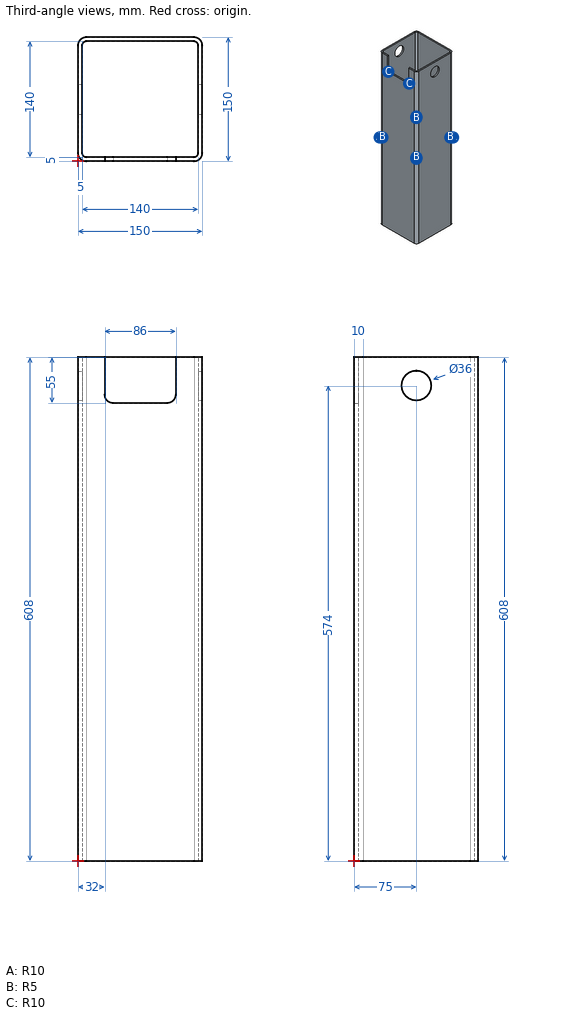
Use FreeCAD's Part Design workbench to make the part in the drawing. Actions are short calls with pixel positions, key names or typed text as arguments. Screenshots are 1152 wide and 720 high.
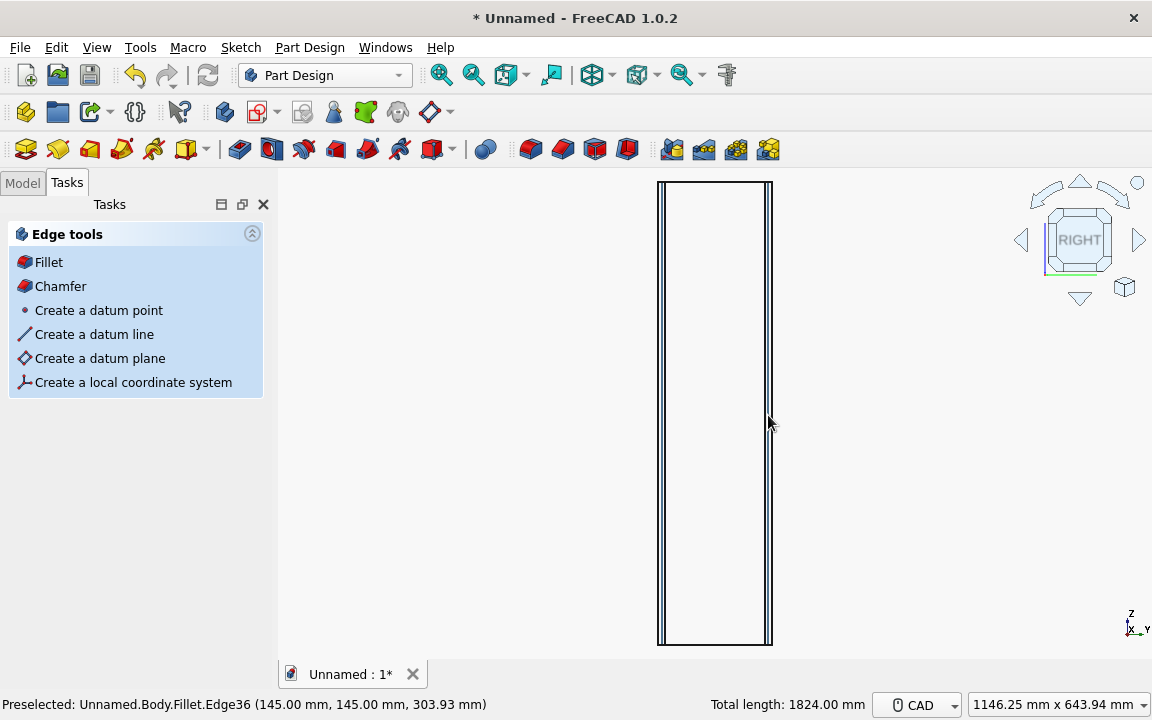
key(5)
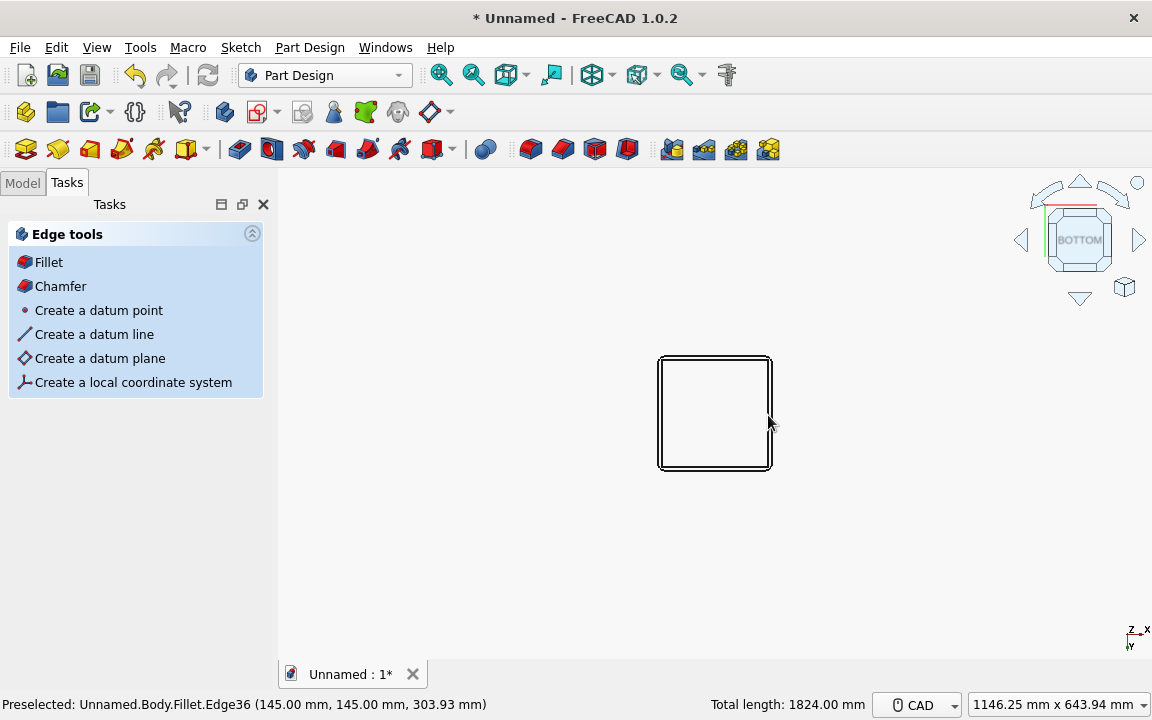
key(v)
key(f)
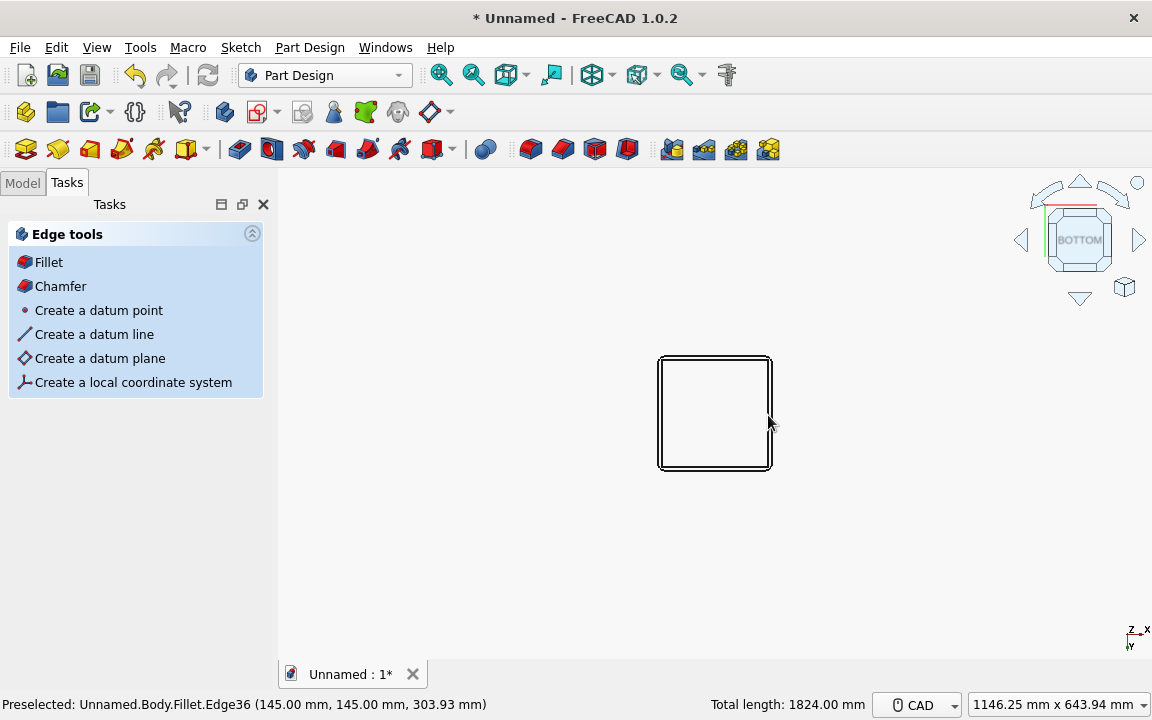
scroll(662, 466, up, 6)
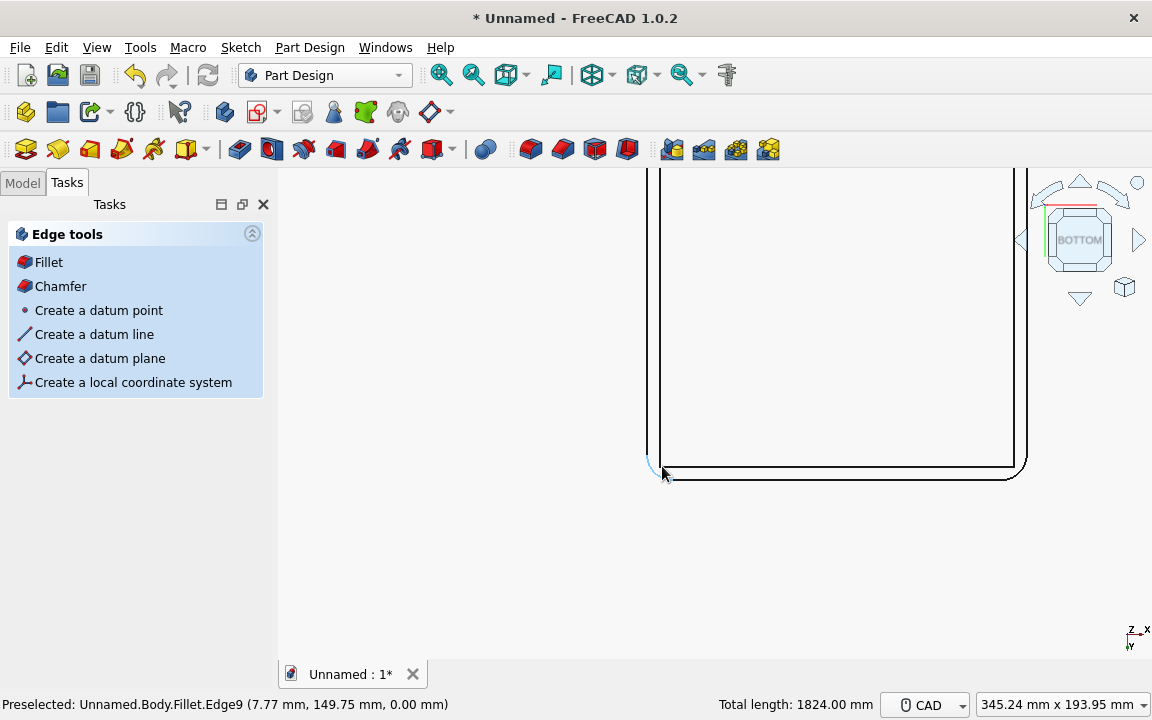
key(v)
key(f)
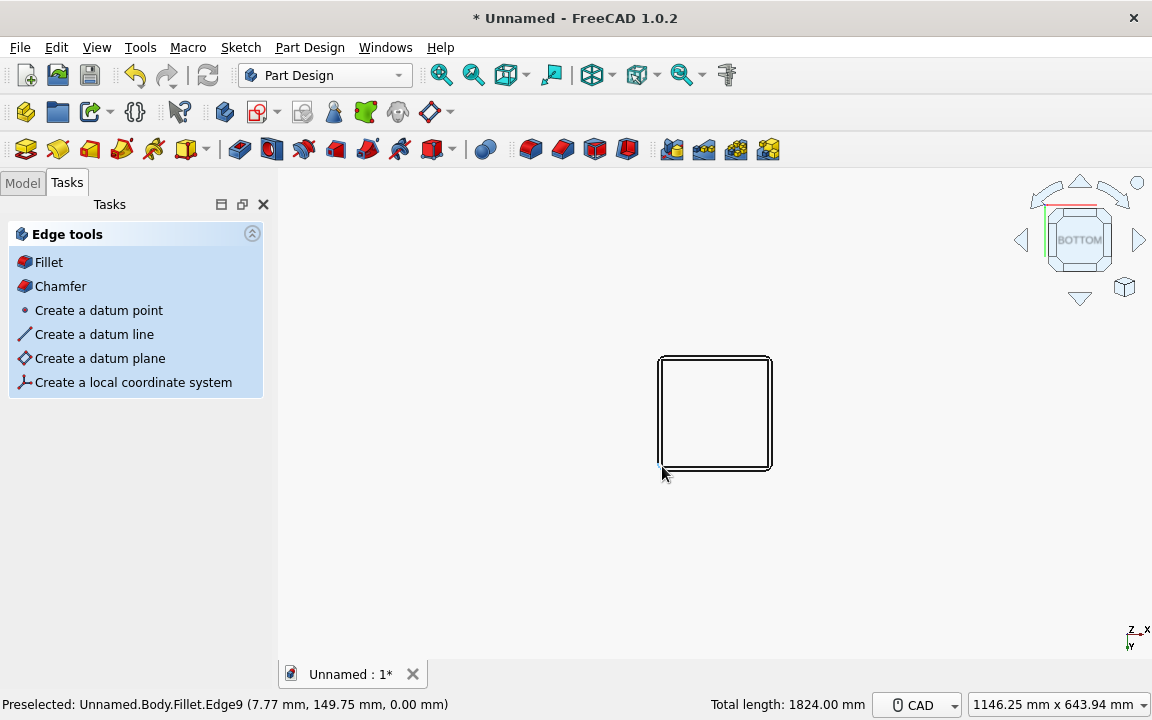
key(4)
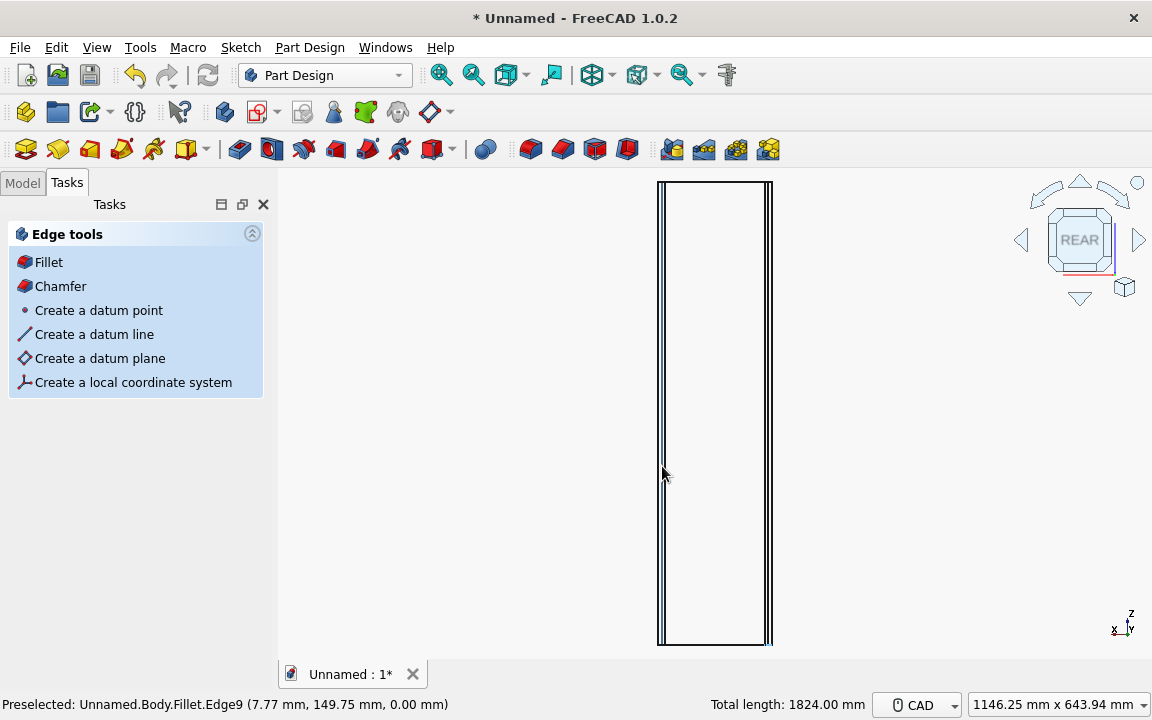
scroll(768, 413, up, 6)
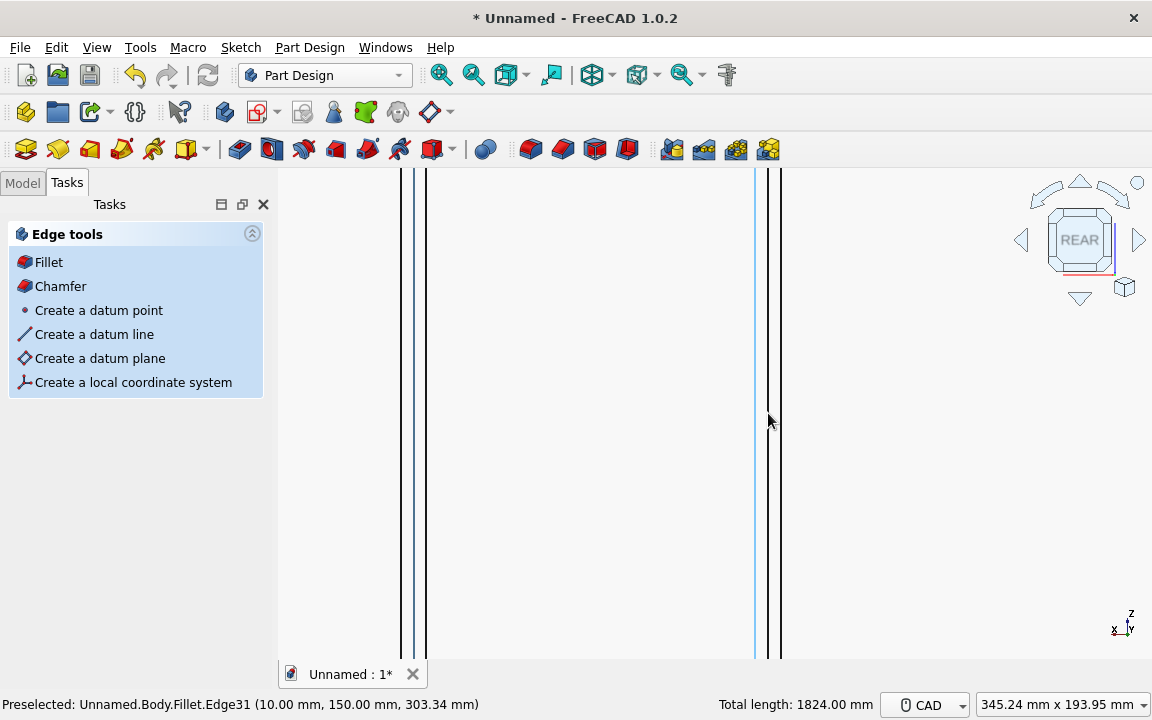
click(768, 413, ctrl)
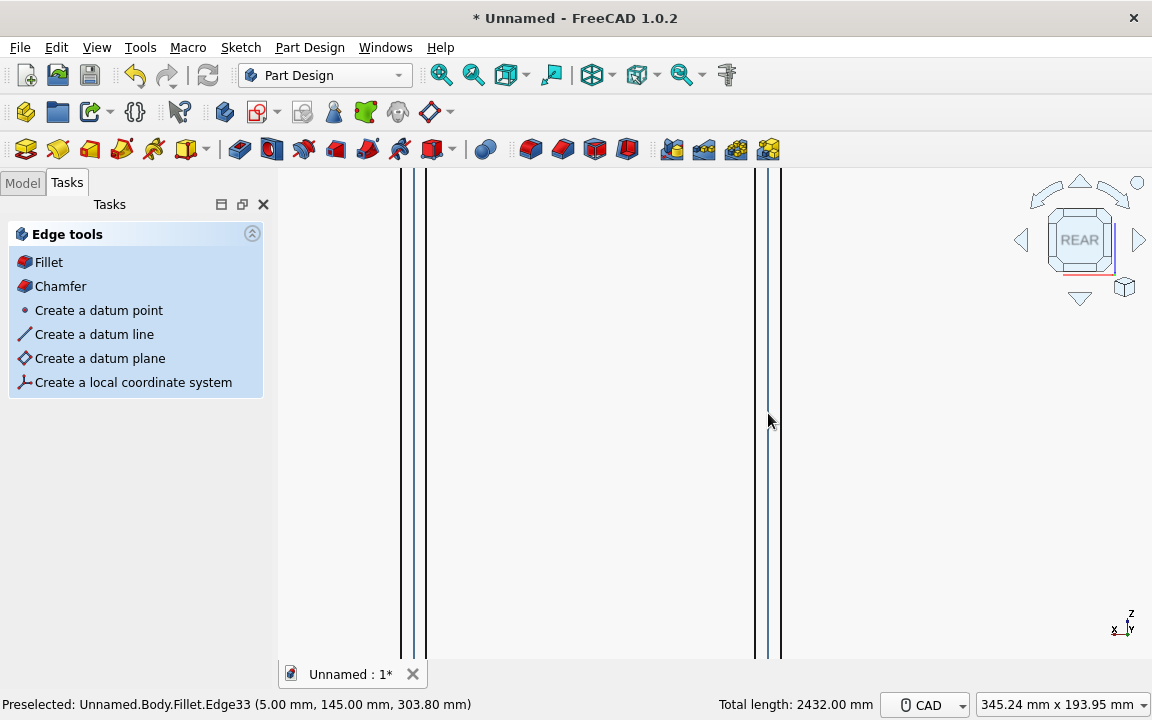
key(v)
key(1)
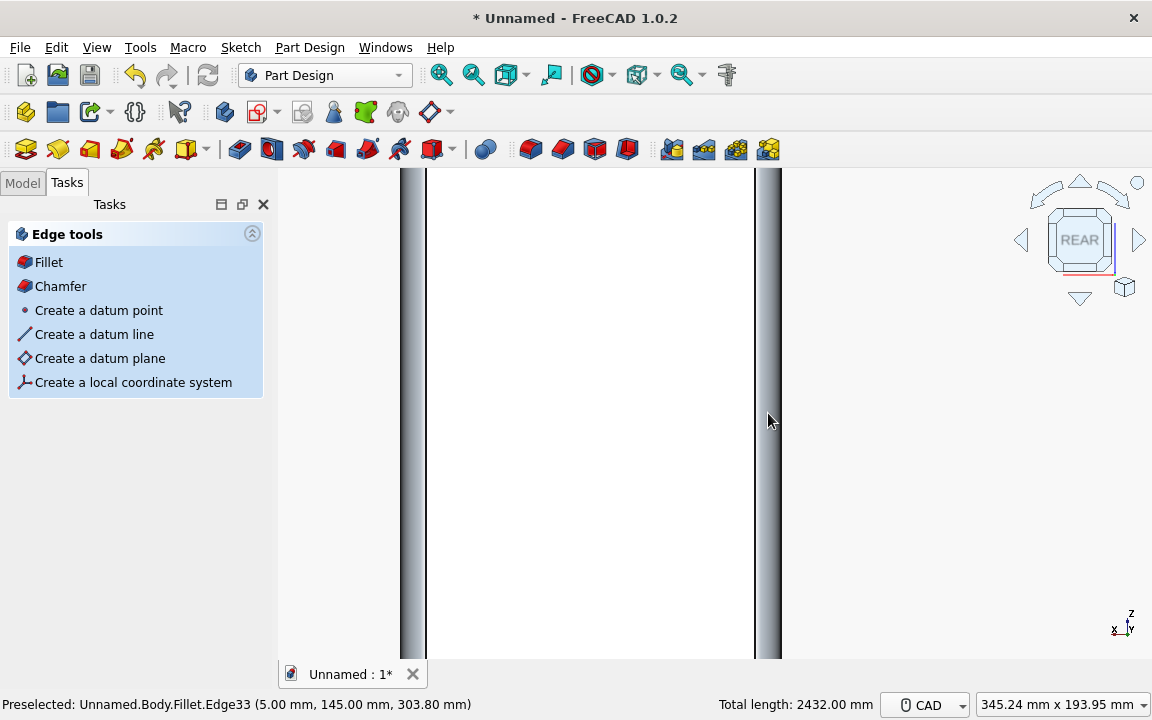
click(532, 150)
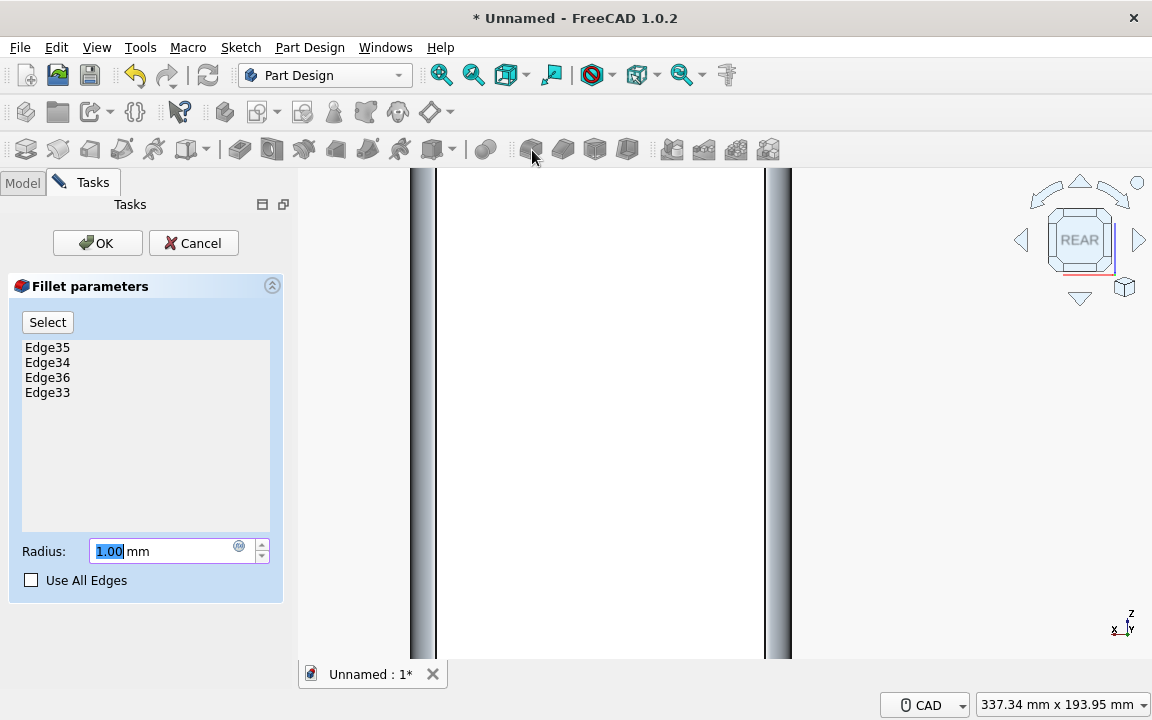
text(5)
key(Tab)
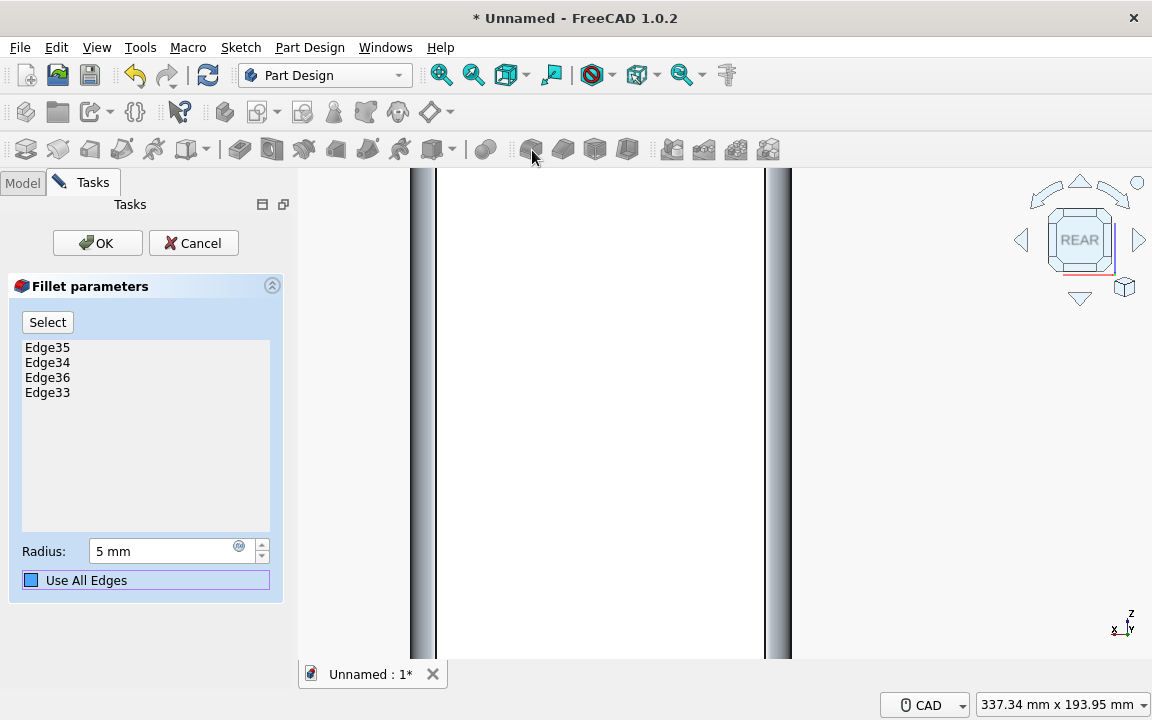
click(98, 243)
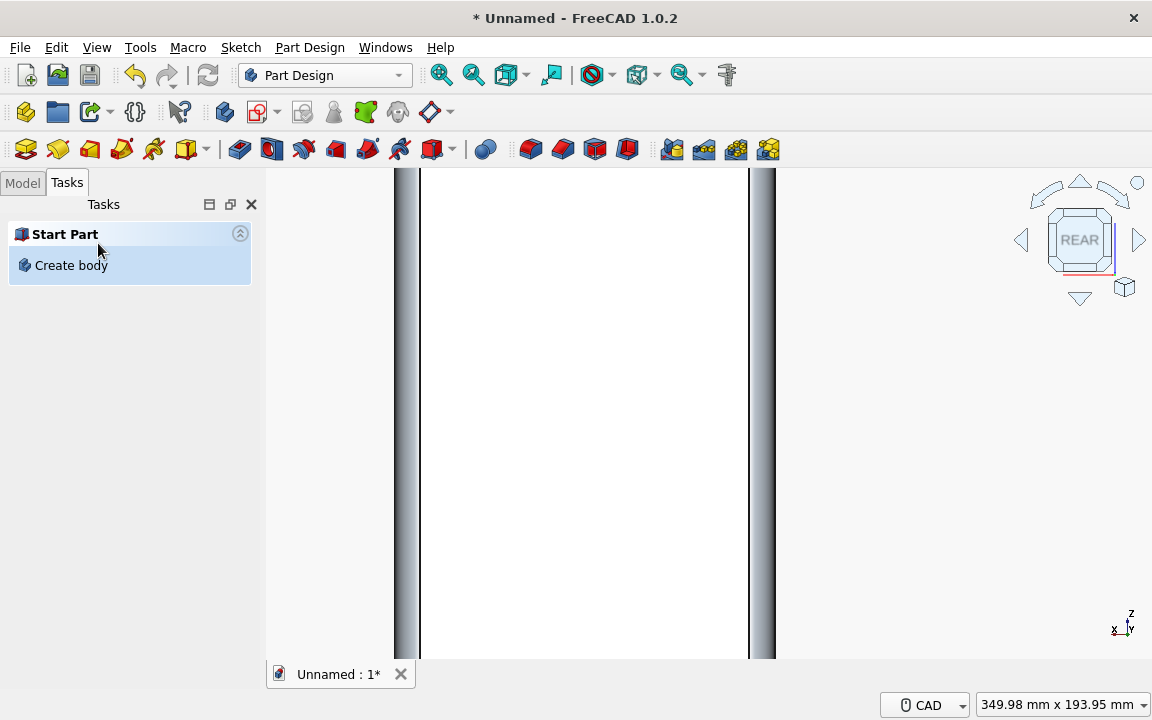
key(v)
key(f)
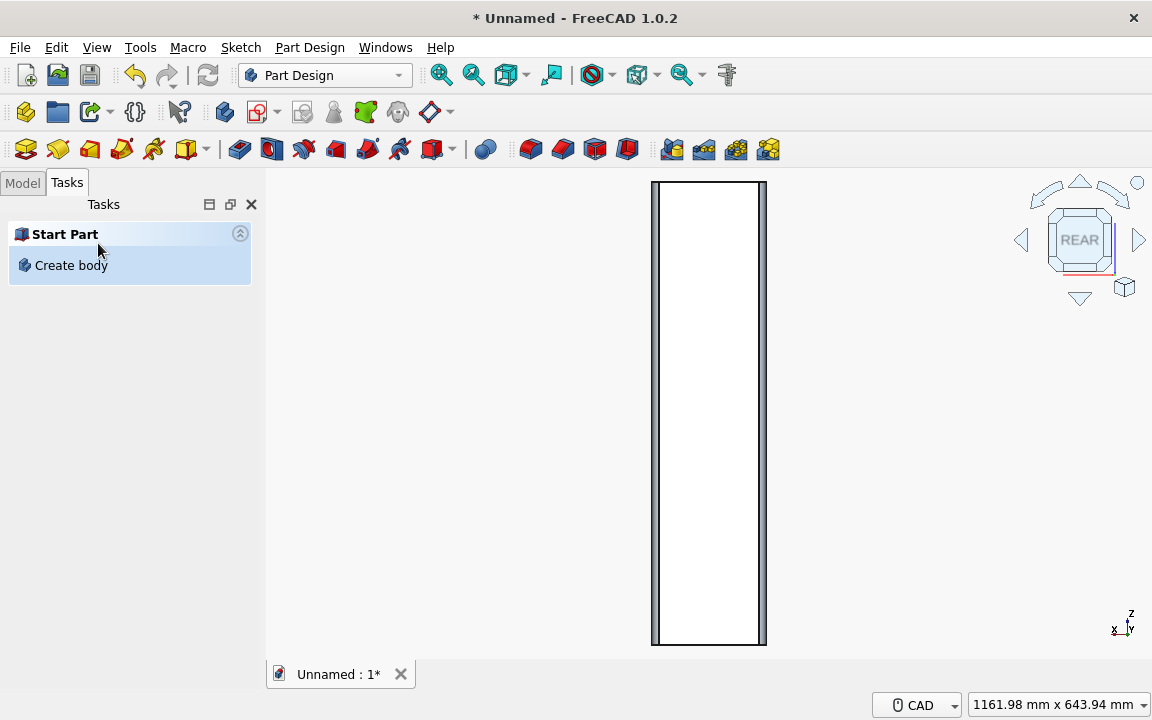
key(6)